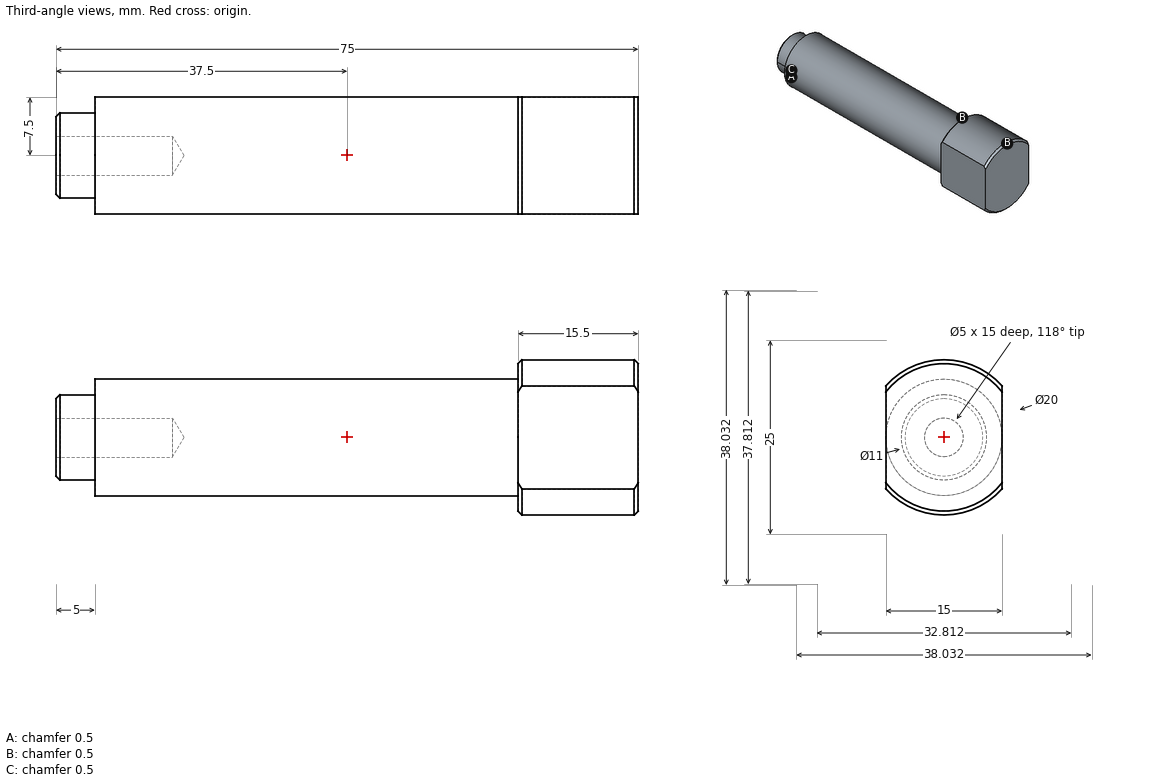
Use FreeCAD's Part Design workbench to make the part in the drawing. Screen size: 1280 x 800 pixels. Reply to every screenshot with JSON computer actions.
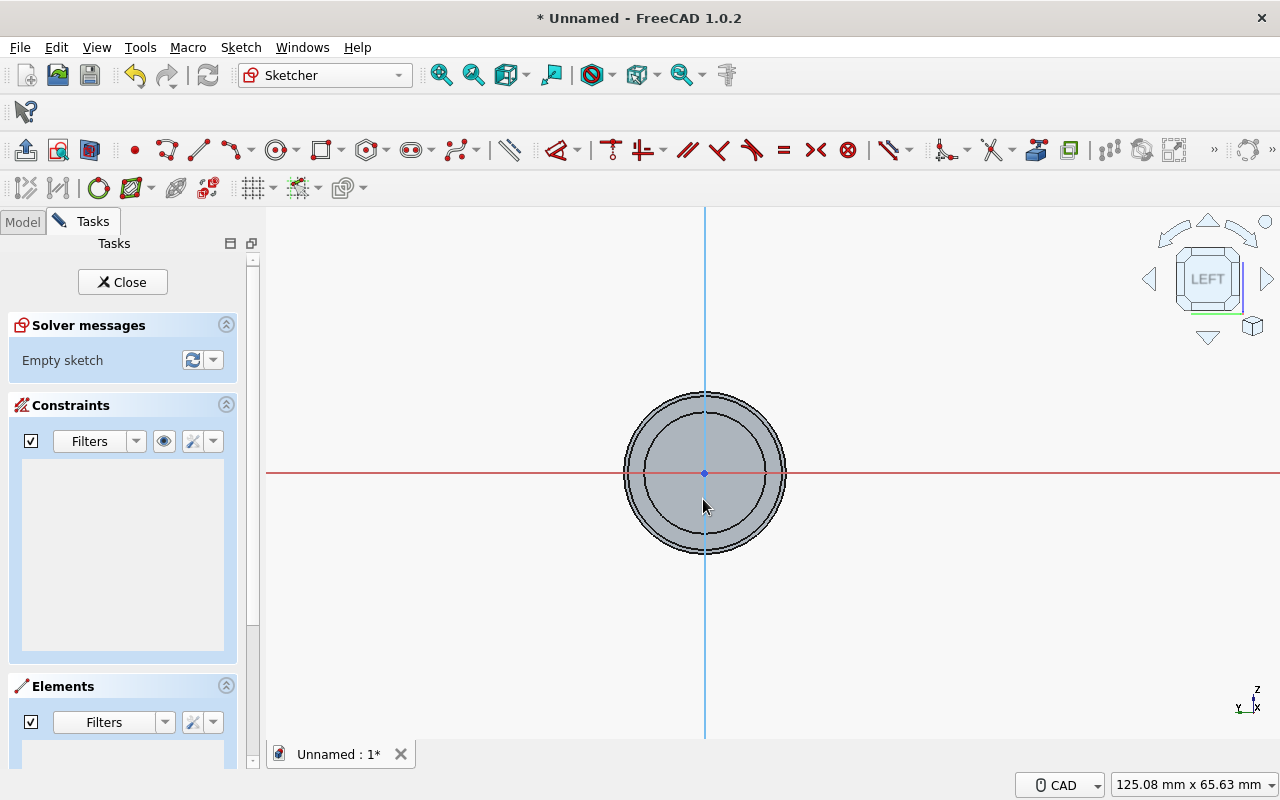
{"action": "left_click", "coordinate": [344, 150]}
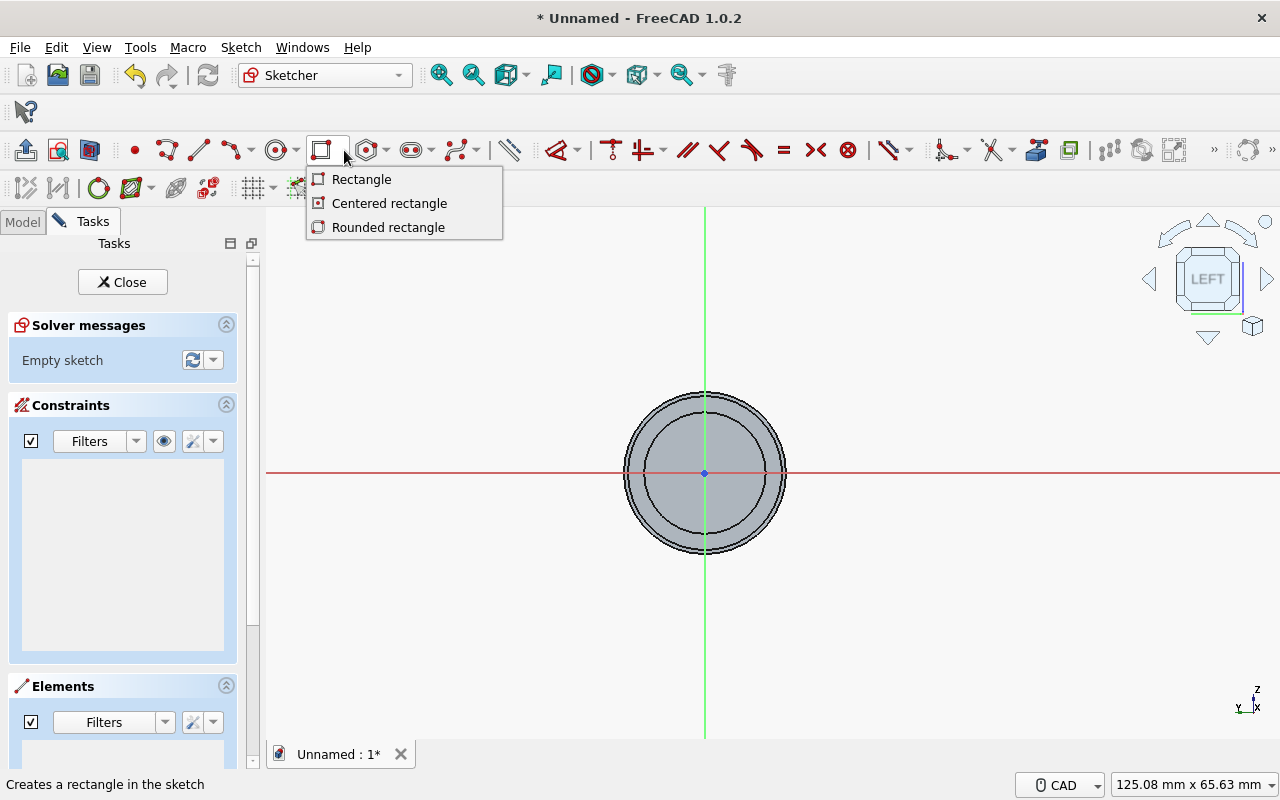
{"action": "left_click", "coordinate": [404, 203]}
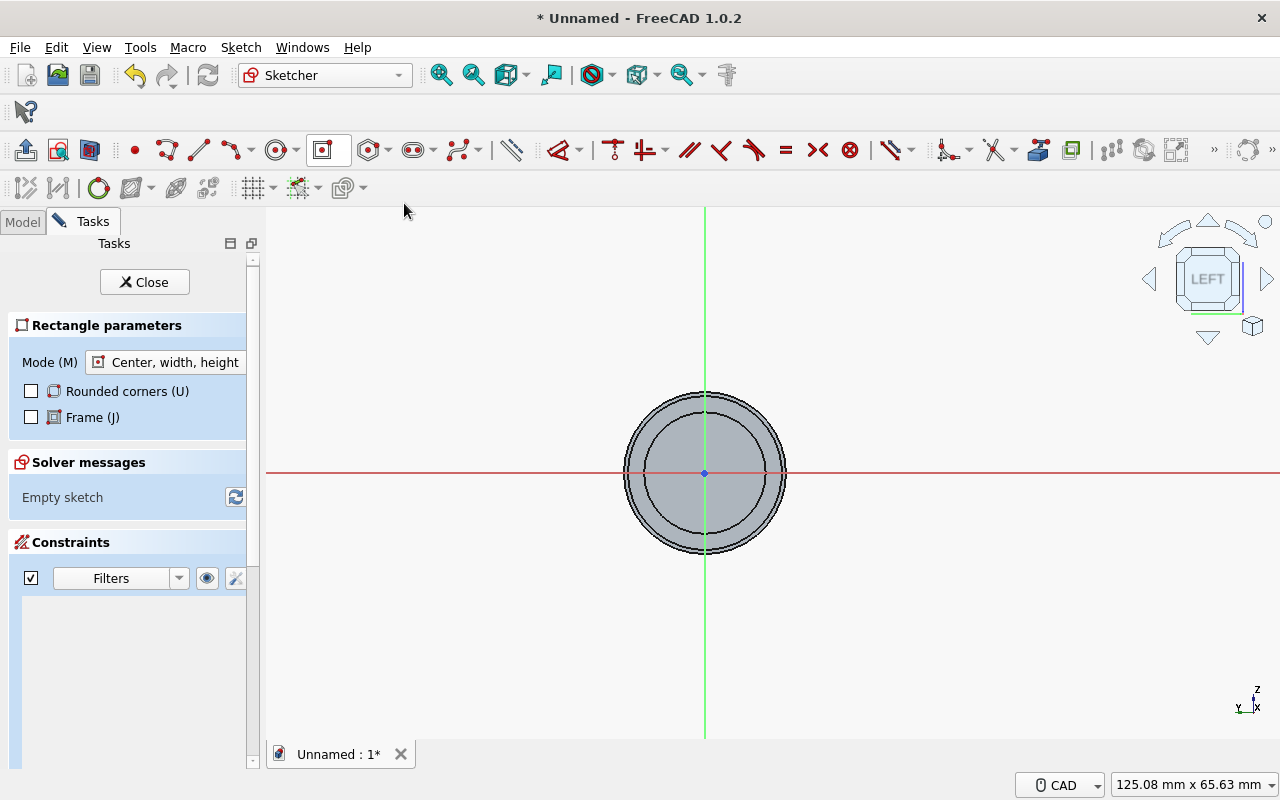
{"action": "left_click", "coordinate": [705, 473]}
{"action": "left_click", "coordinate": [859, 319]}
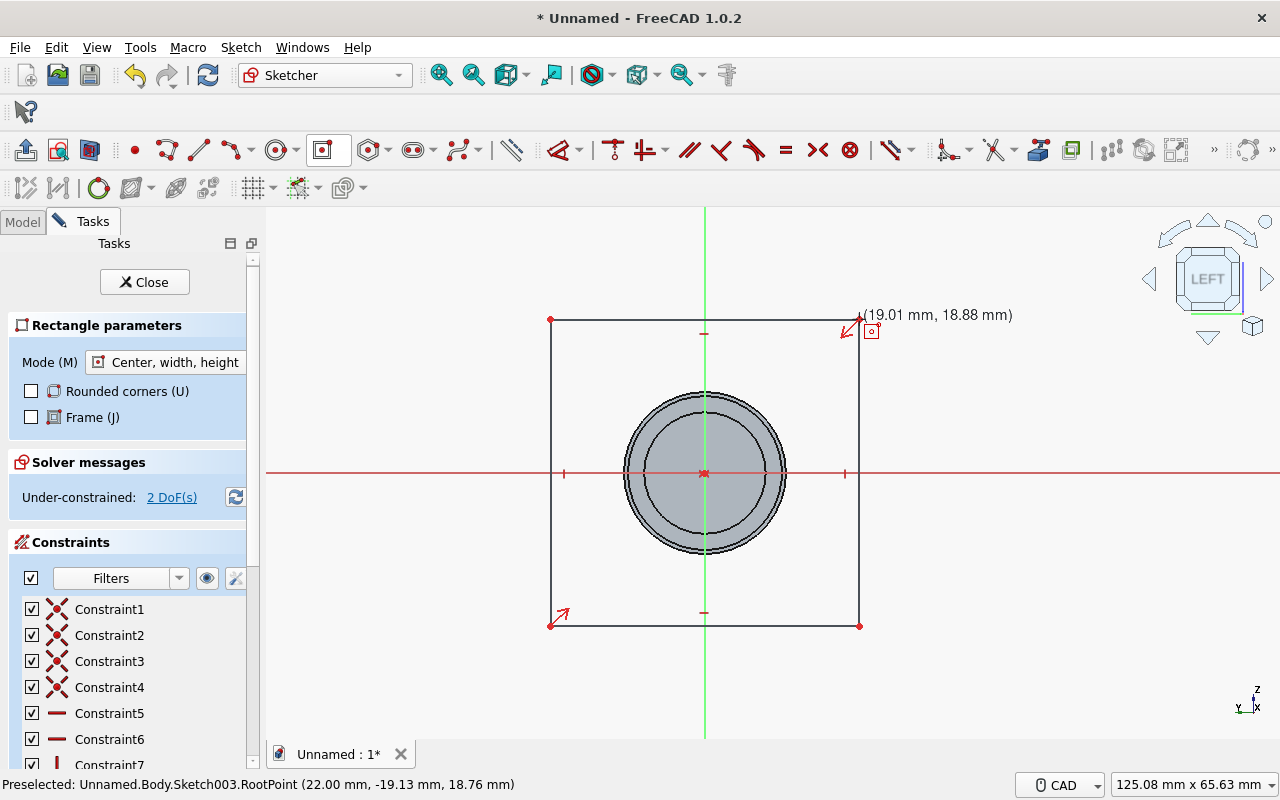
{"action": "left_click", "coordinate": [705, 473]}
{"action": "left_click", "coordinate": [766, 372]}
{"action": "key", "text": "Escape"}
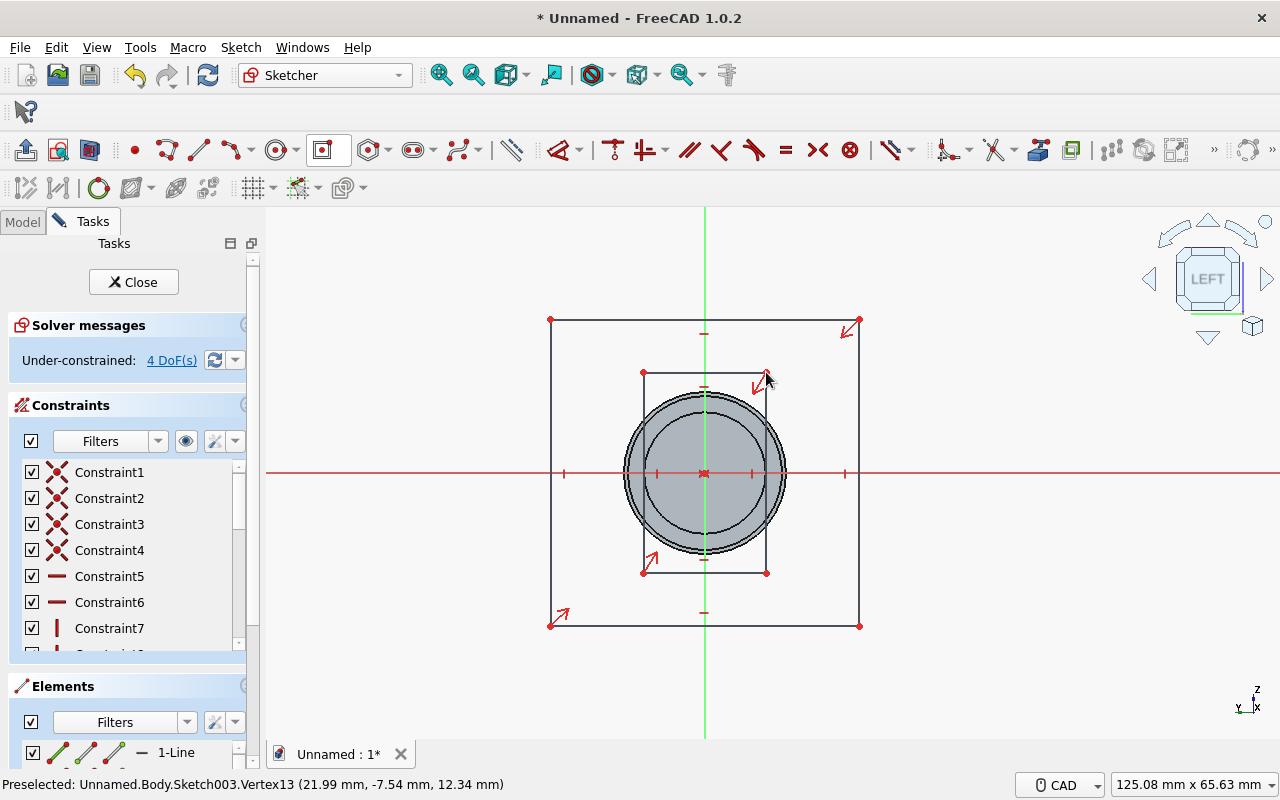
{"action": "left_click", "coordinate": [558, 150]}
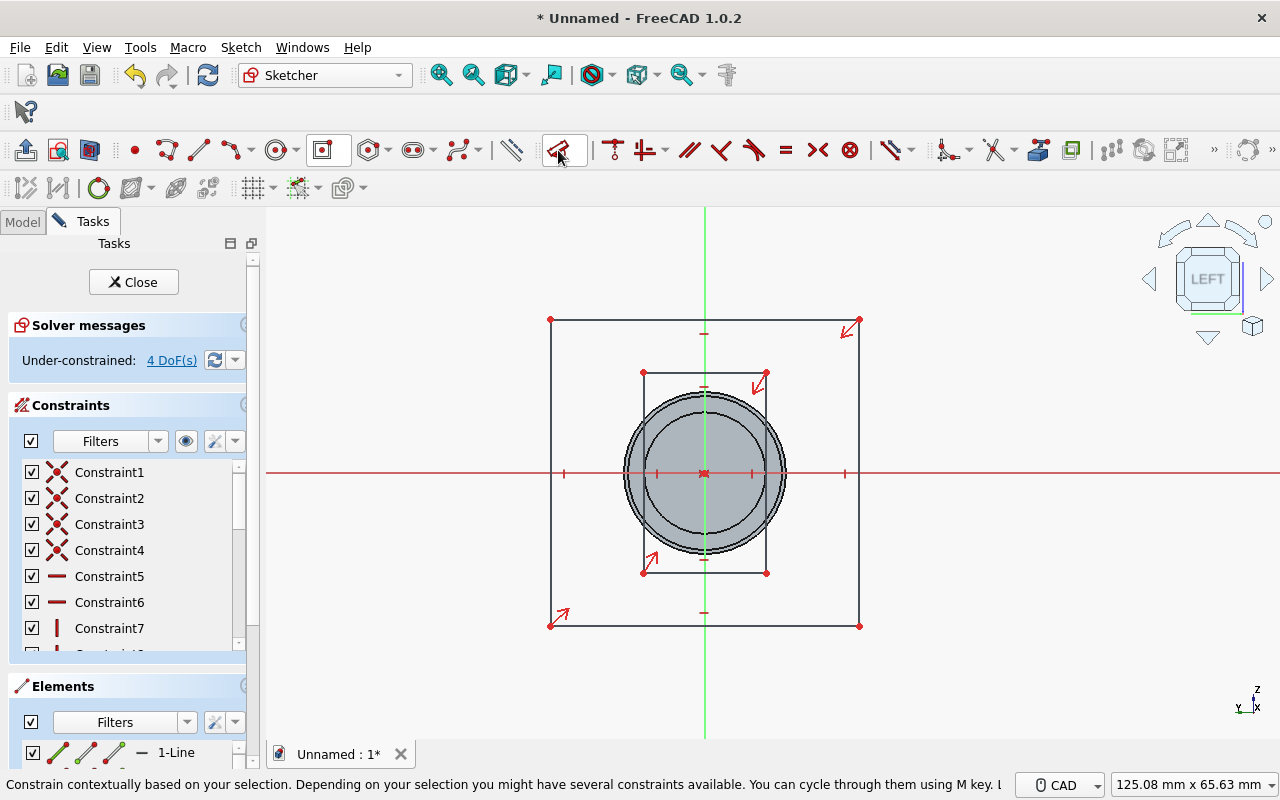
{"action": "left_click", "coordinate": [680, 573]}
{"action": "left_click", "coordinate": [677, 607]}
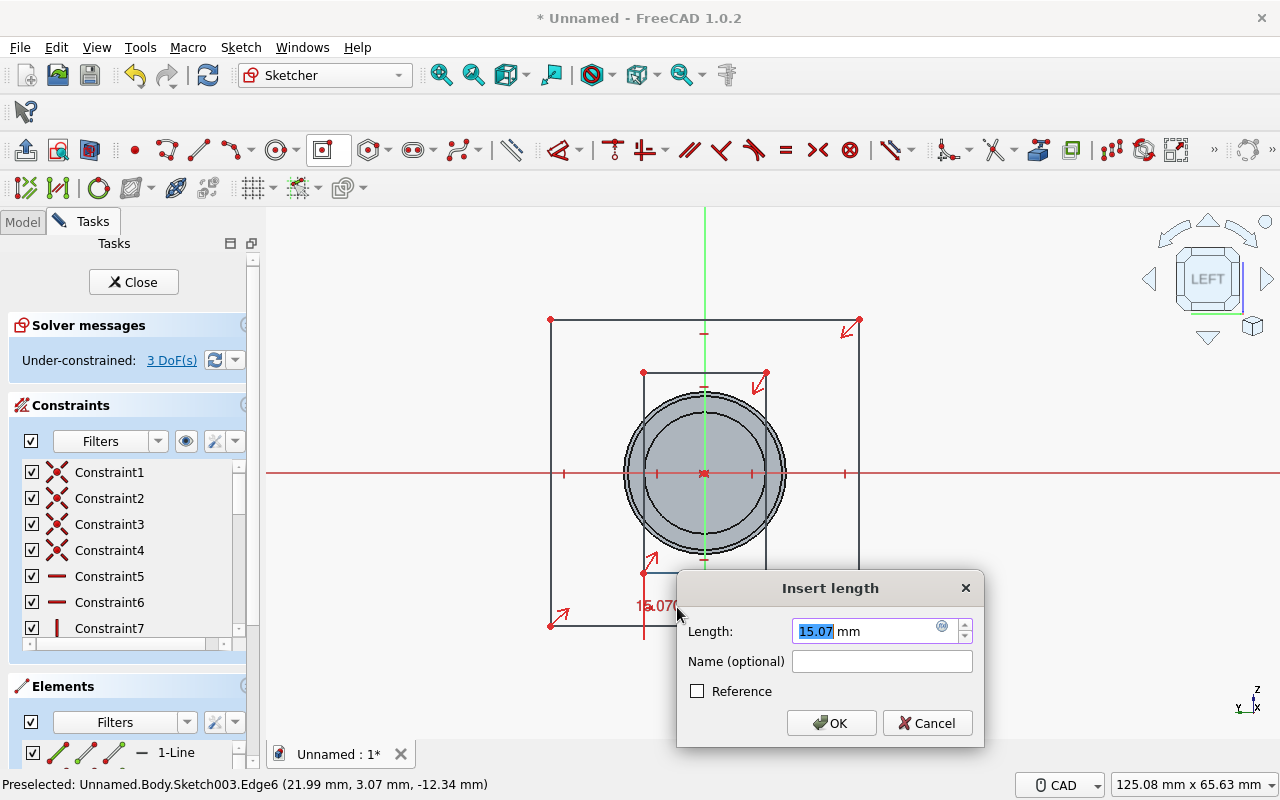
{"action": "type", "text": "15"}
{"action": "key", "text": "Return"}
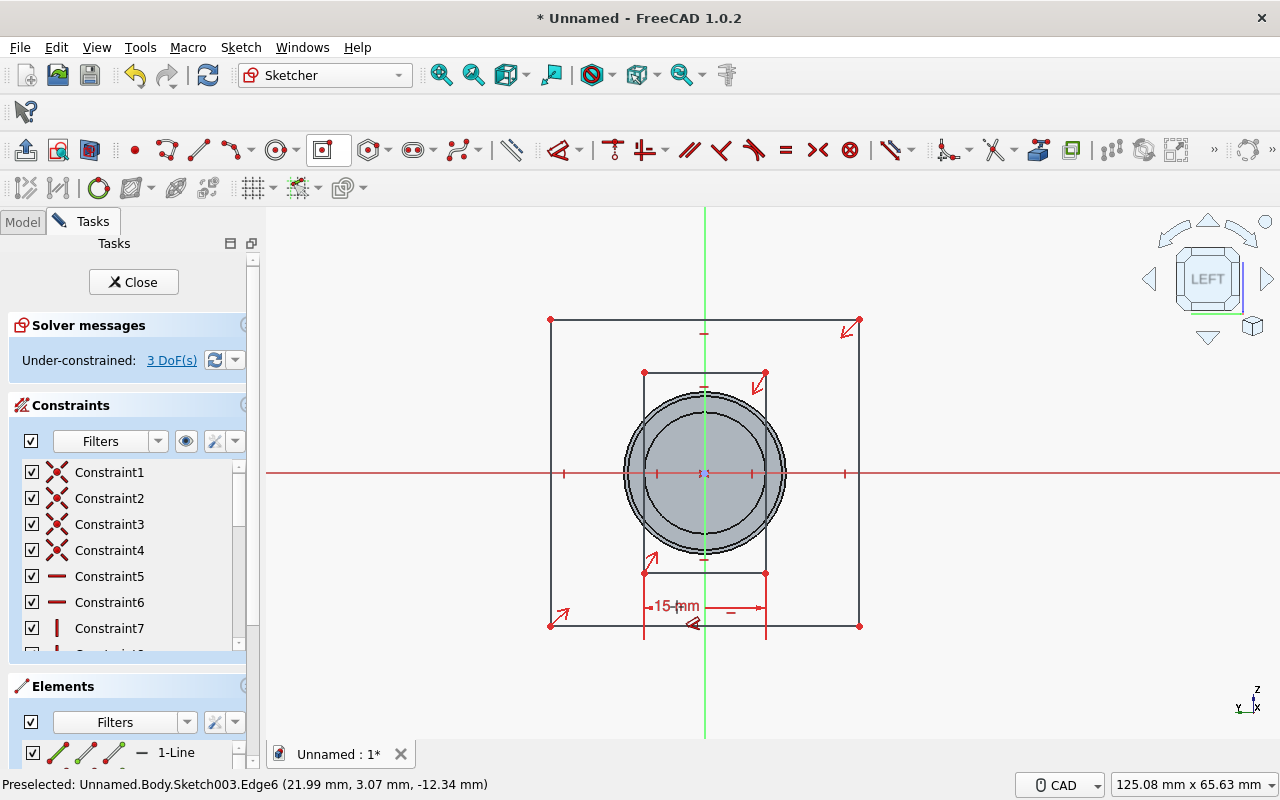
{"action": "left_click", "coordinate": [766, 513]}
{"action": "left_click", "coordinate": [800, 427]}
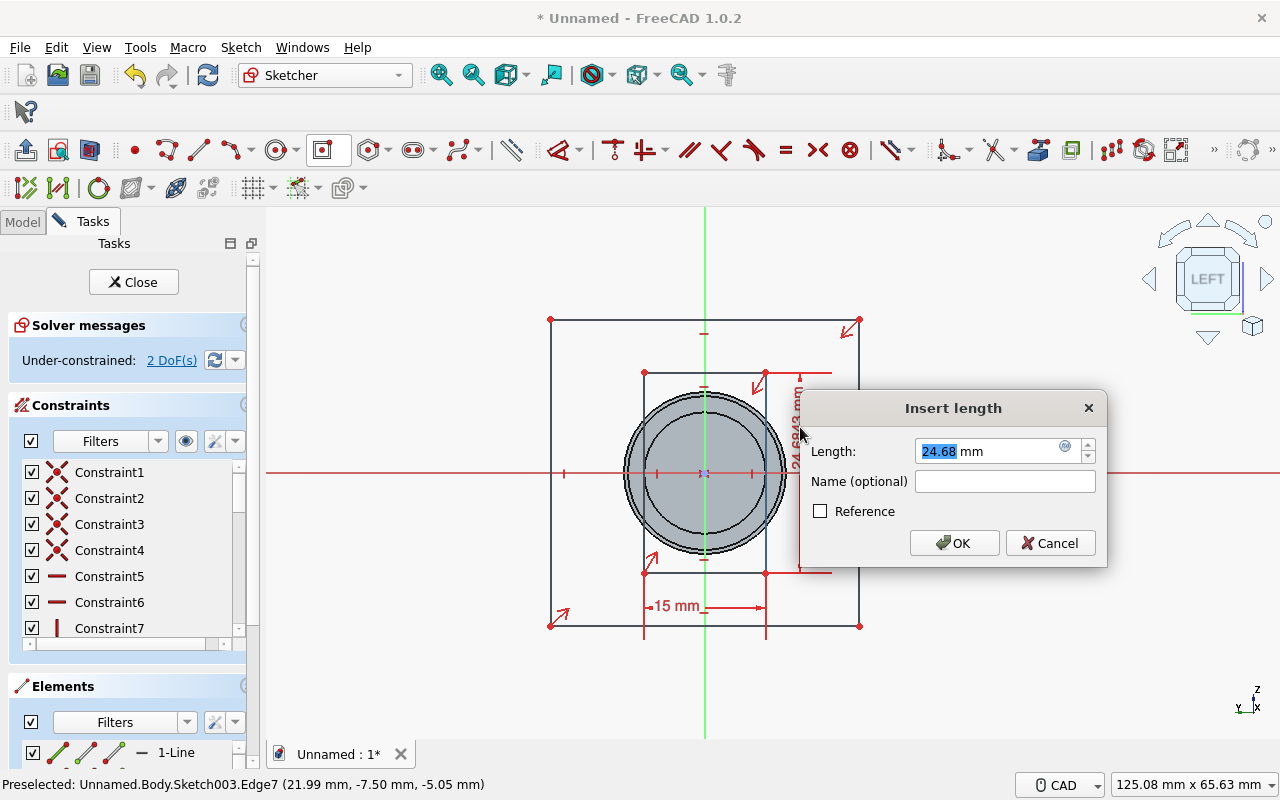
{"action": "type", "text": "25"}
{"action": "key", "text": "Return"}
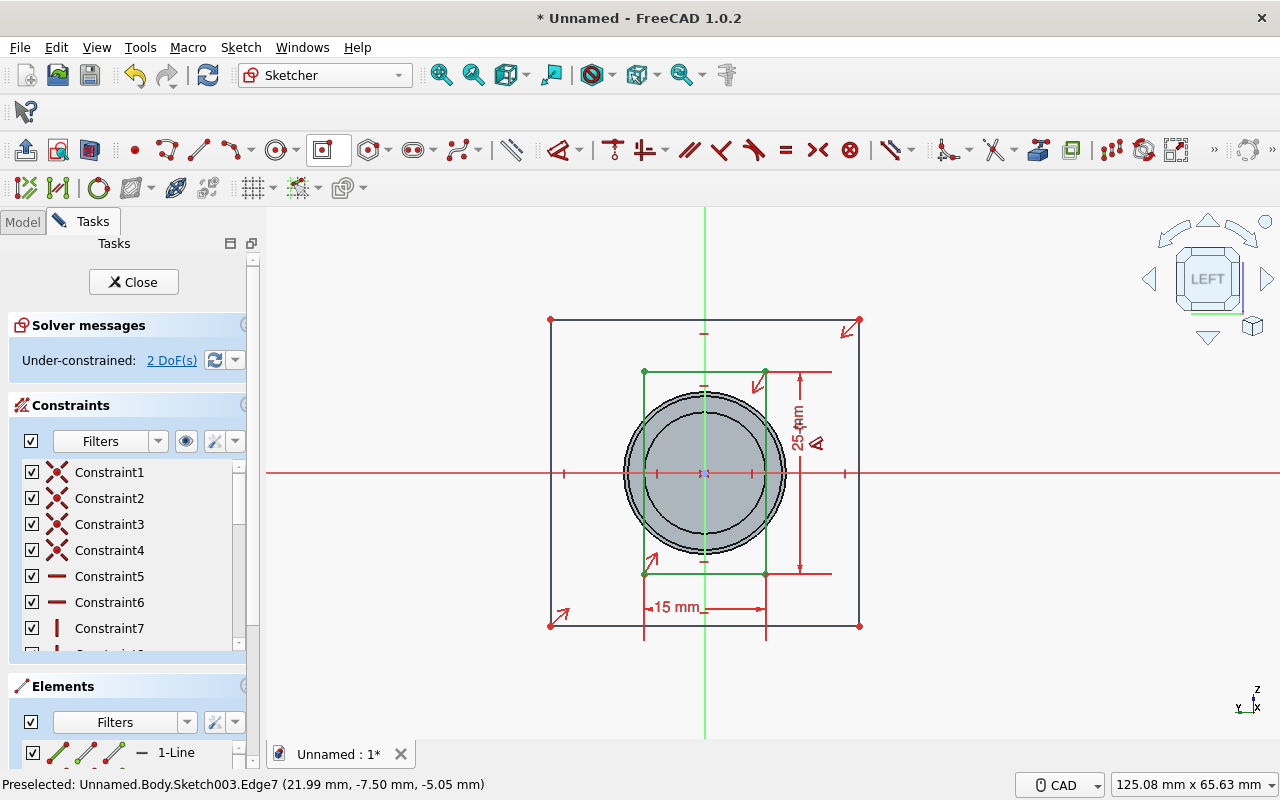
{"action": "left_click", "coordinate": [643, 626]}
{"action": "left_click", "coordinate": [634, 660]}